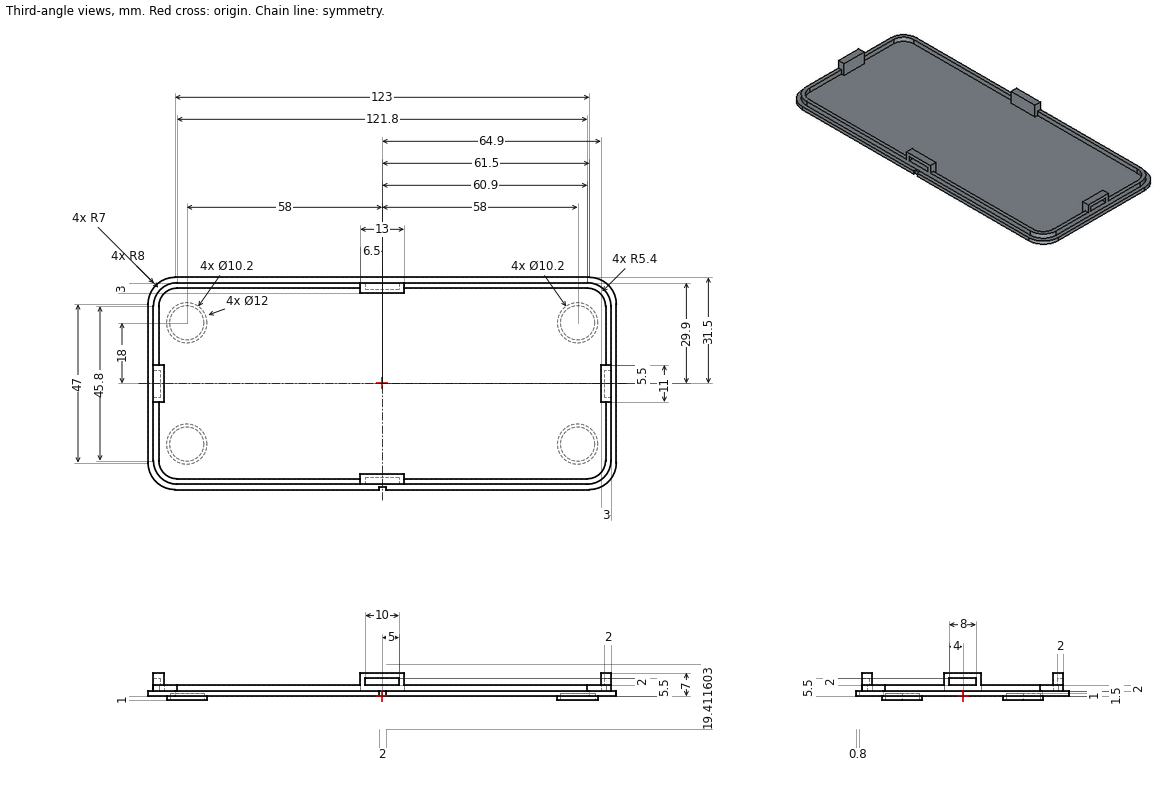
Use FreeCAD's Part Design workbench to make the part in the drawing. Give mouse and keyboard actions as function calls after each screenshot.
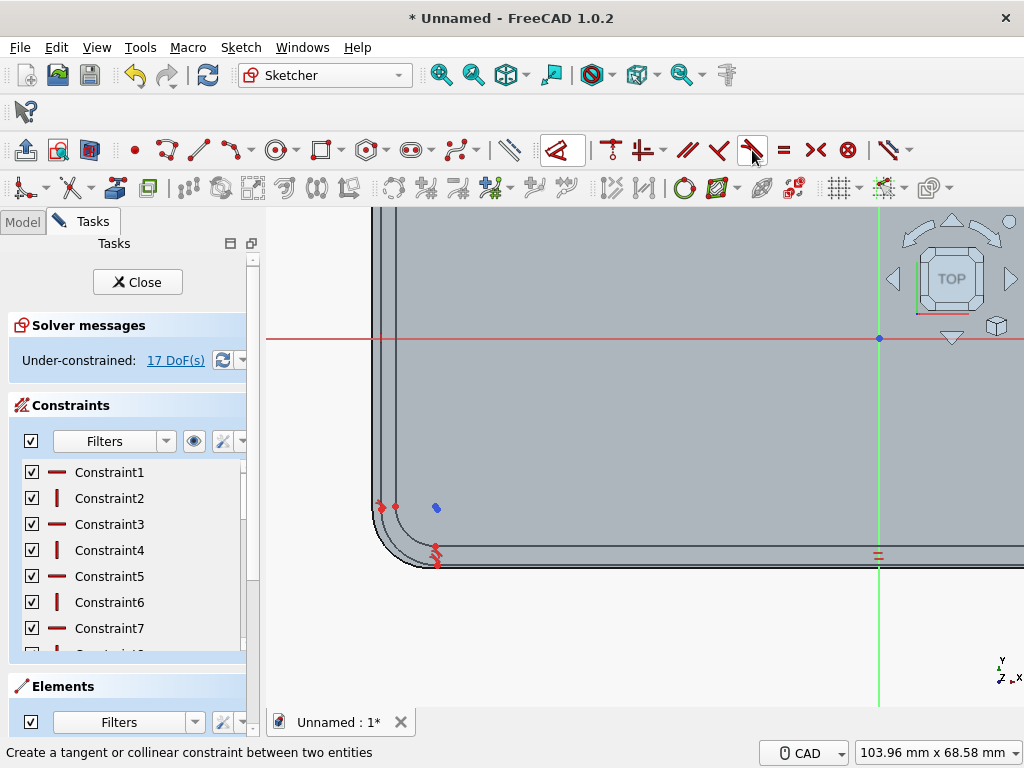
click(396, 406)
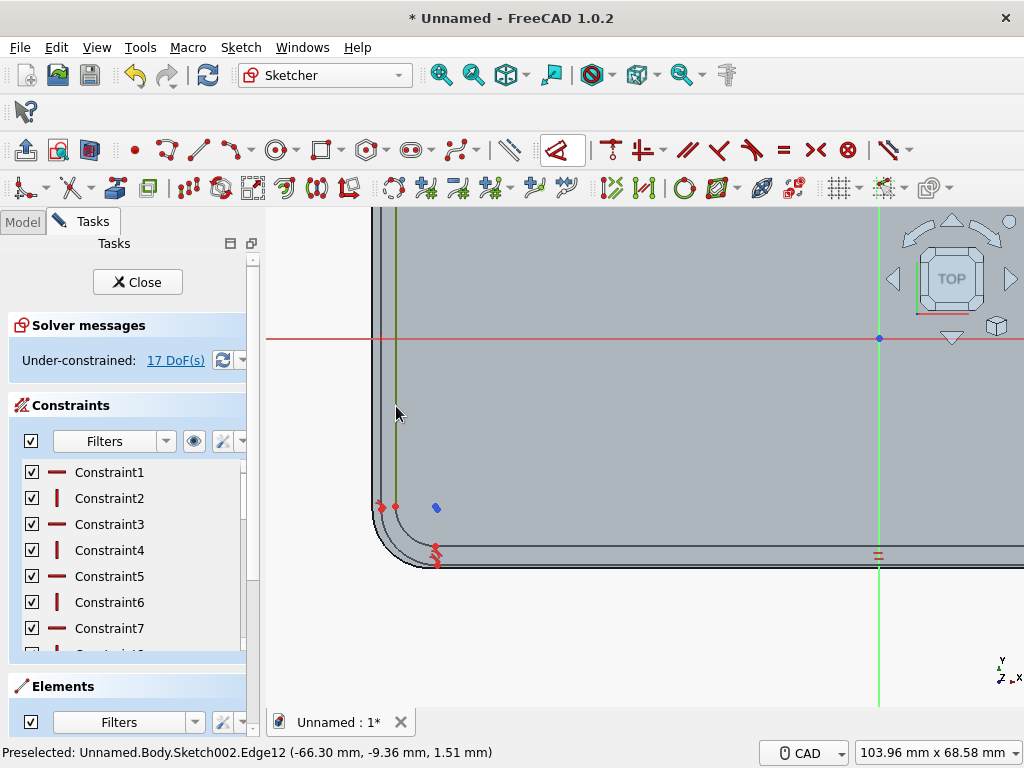
scroll(400, 526, down, 5)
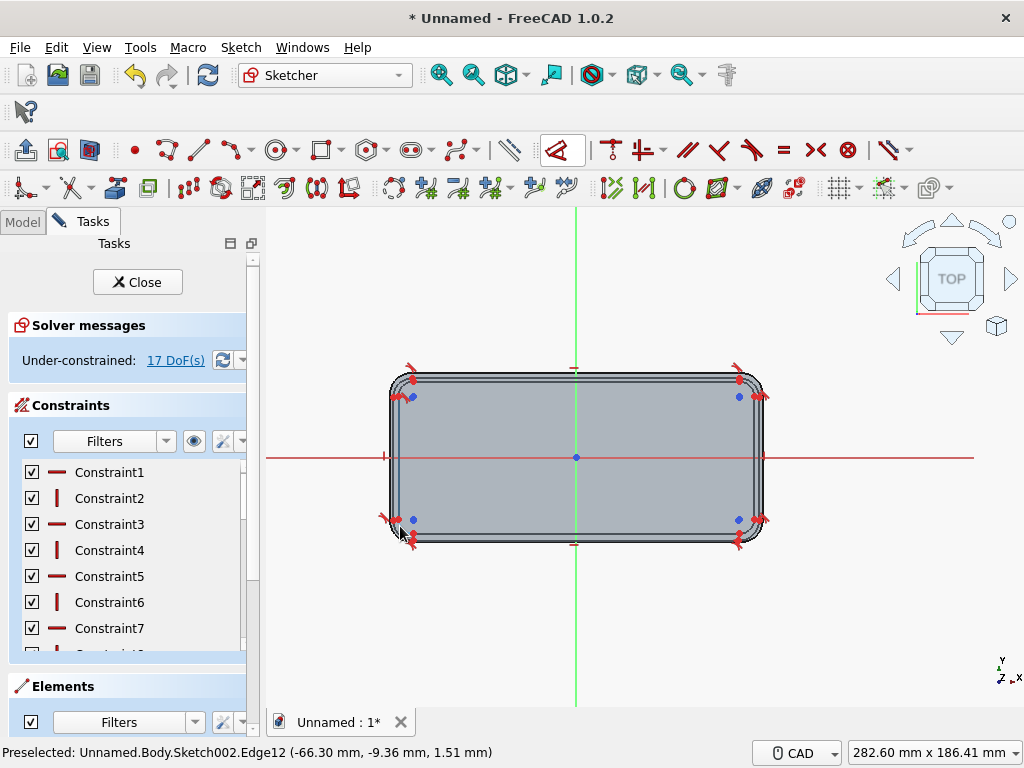
scroll(406, 383, up, 7)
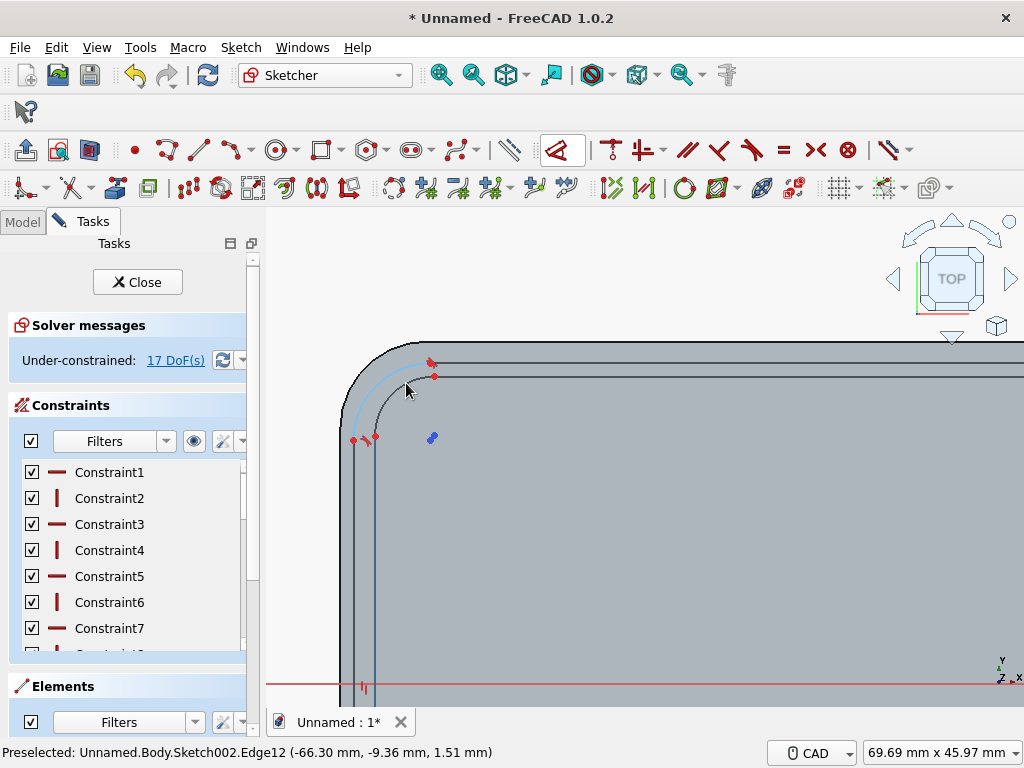
click(407, 383)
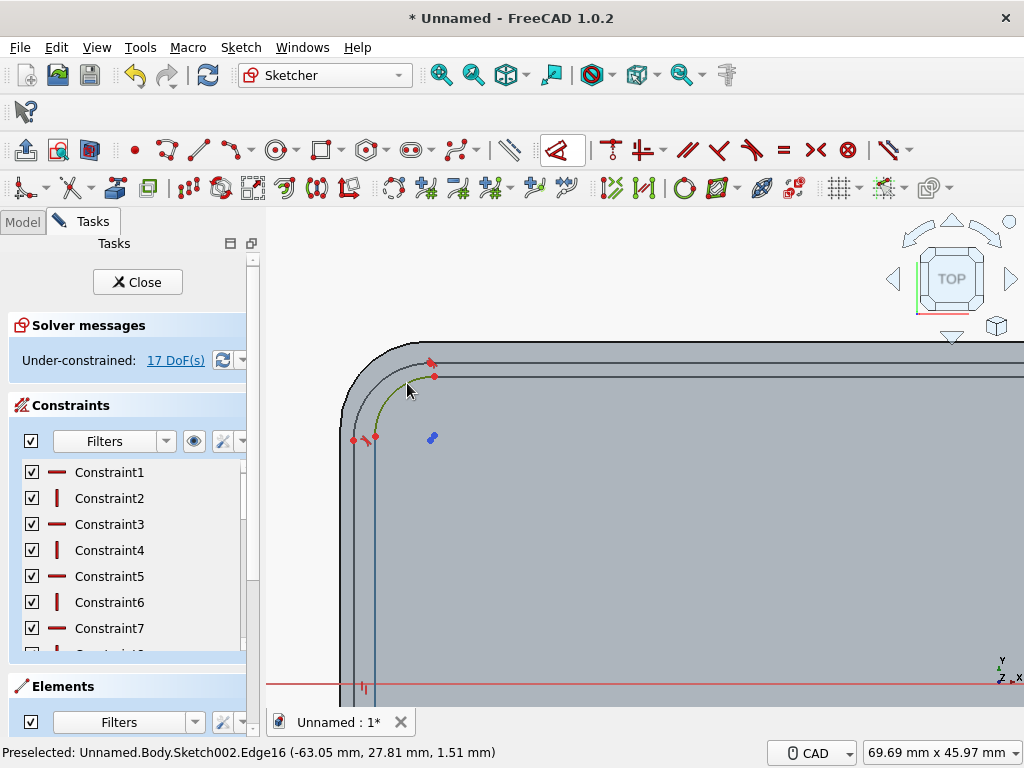
click(752, 150)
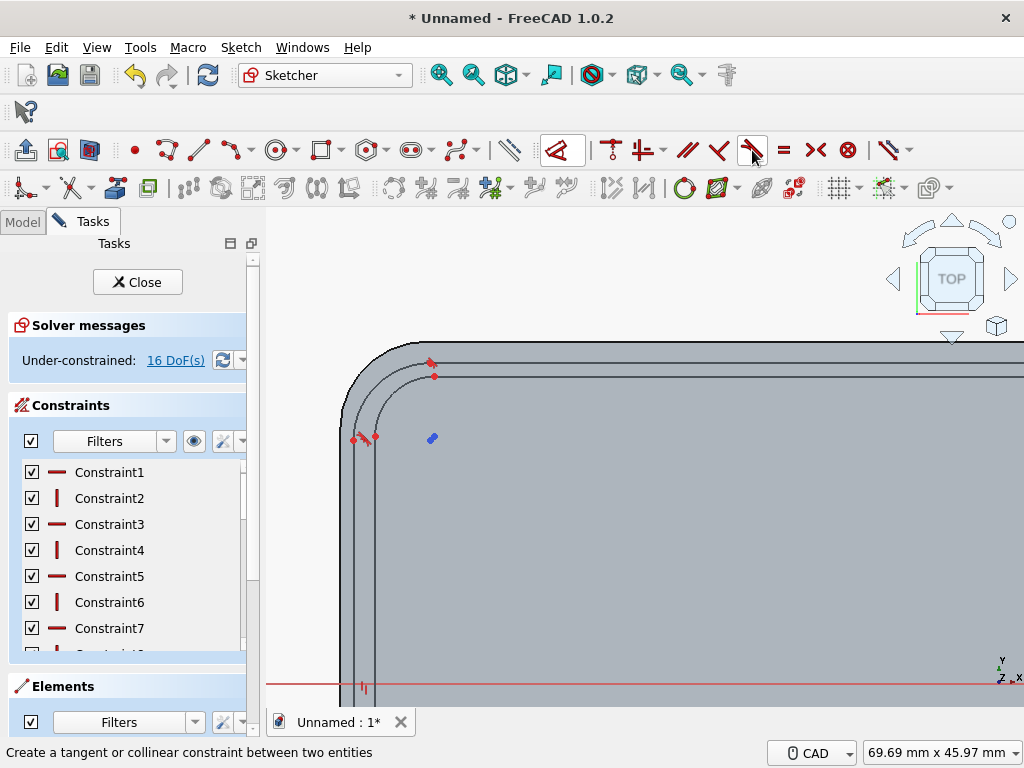
scroll(406, 383, down, 7)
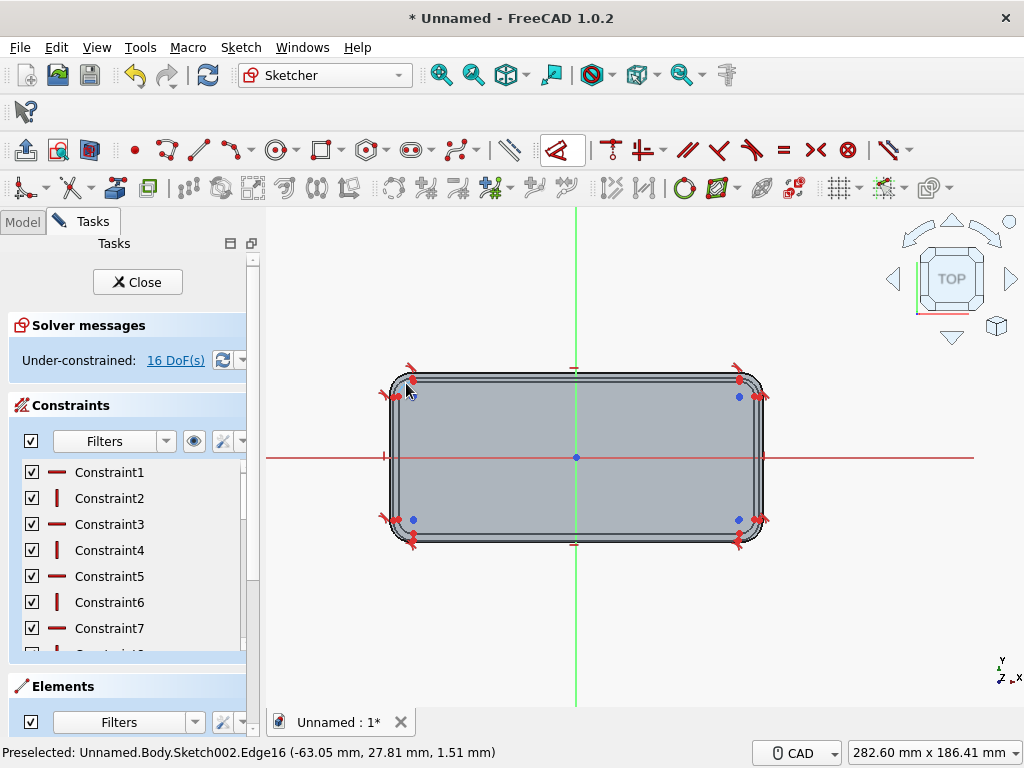
scroll(757, 389, up, 6)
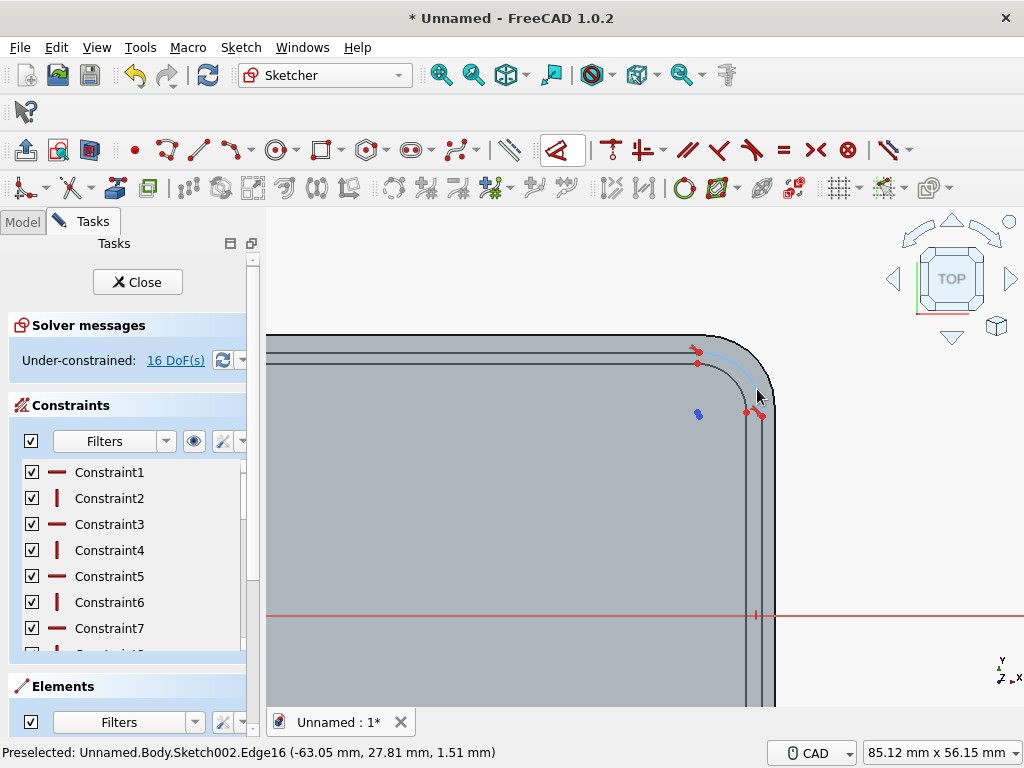
click(755, 387)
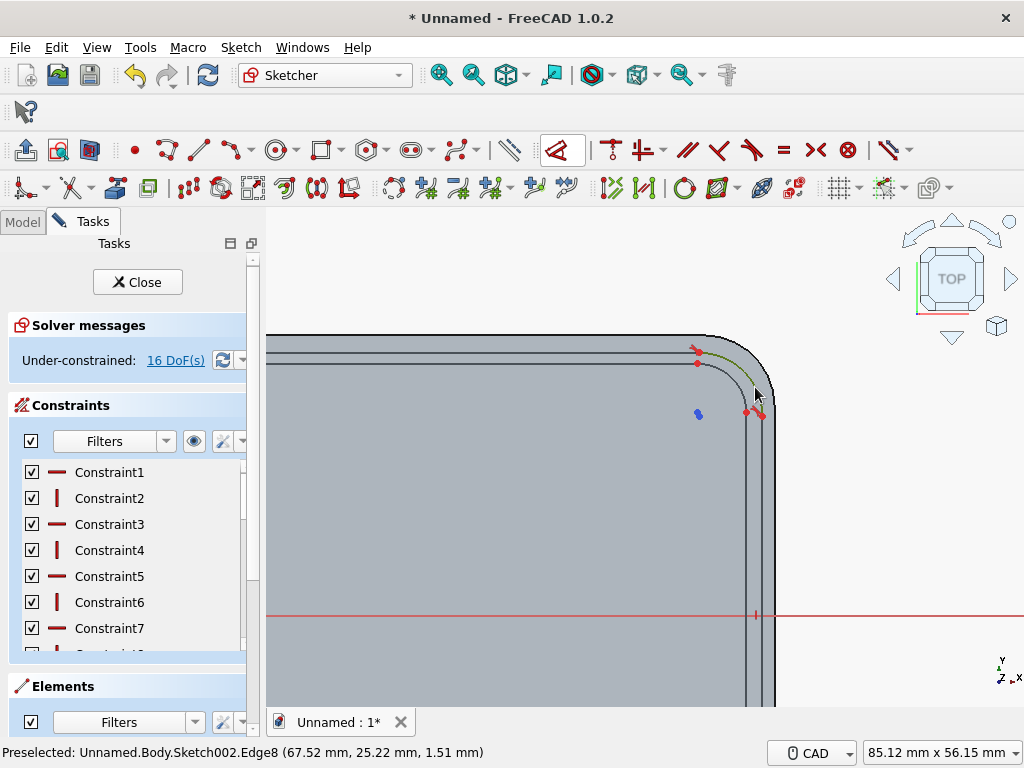
click(741, 390)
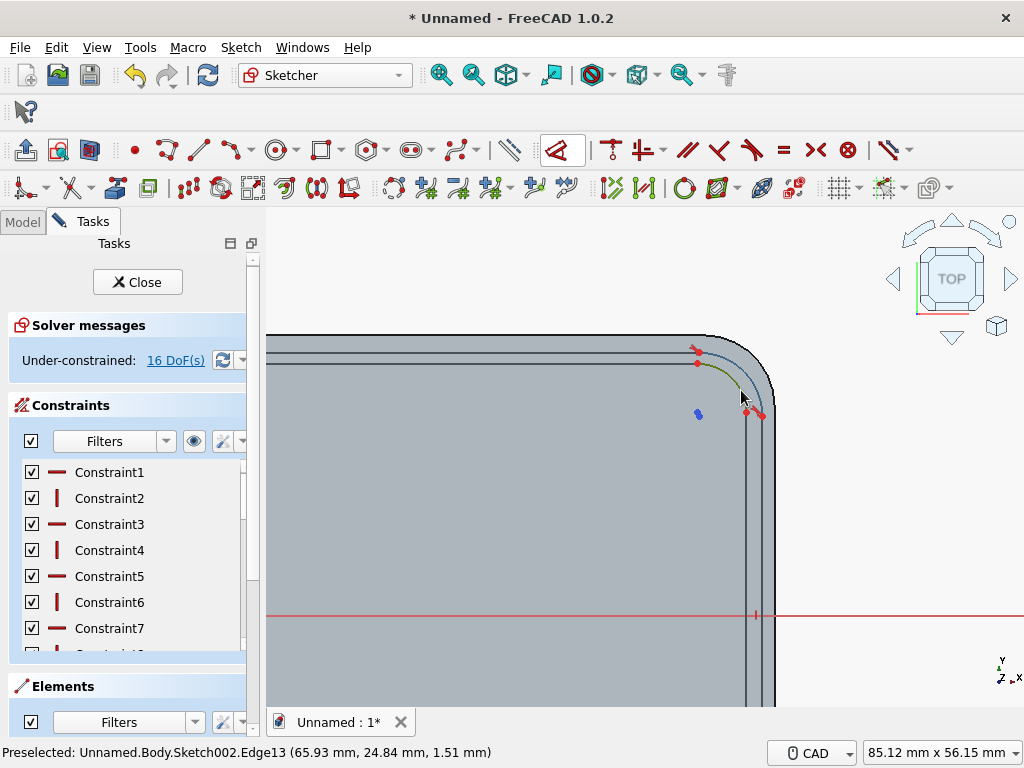
click(612, 150)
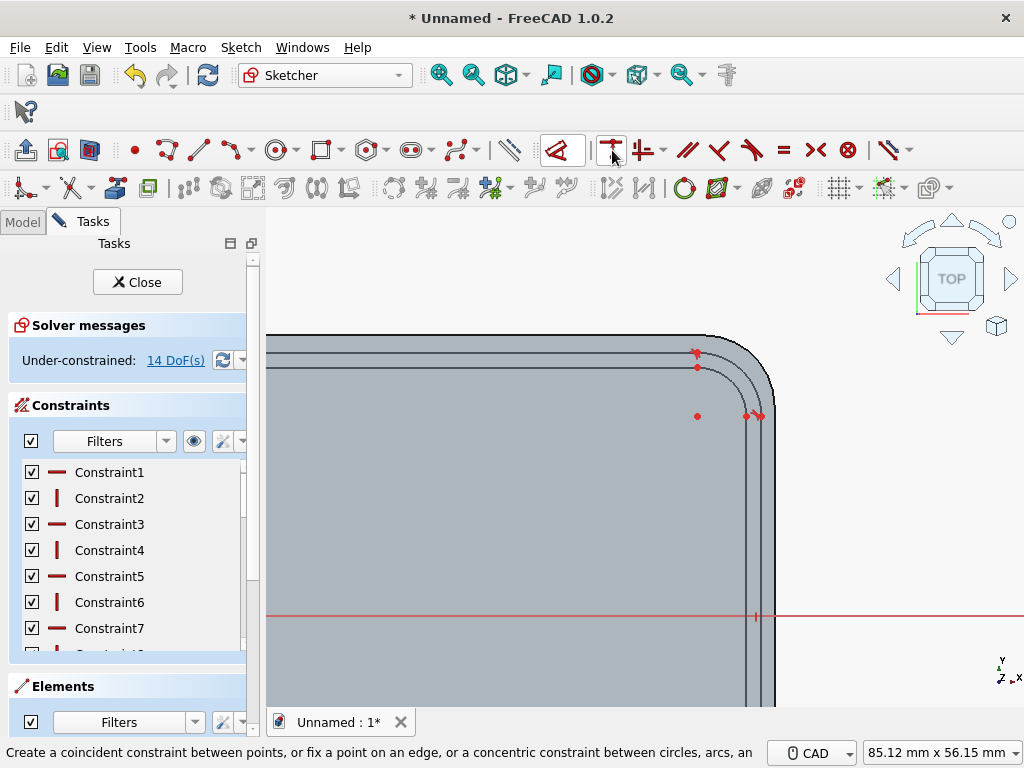
scroll(758, 389, down, 6)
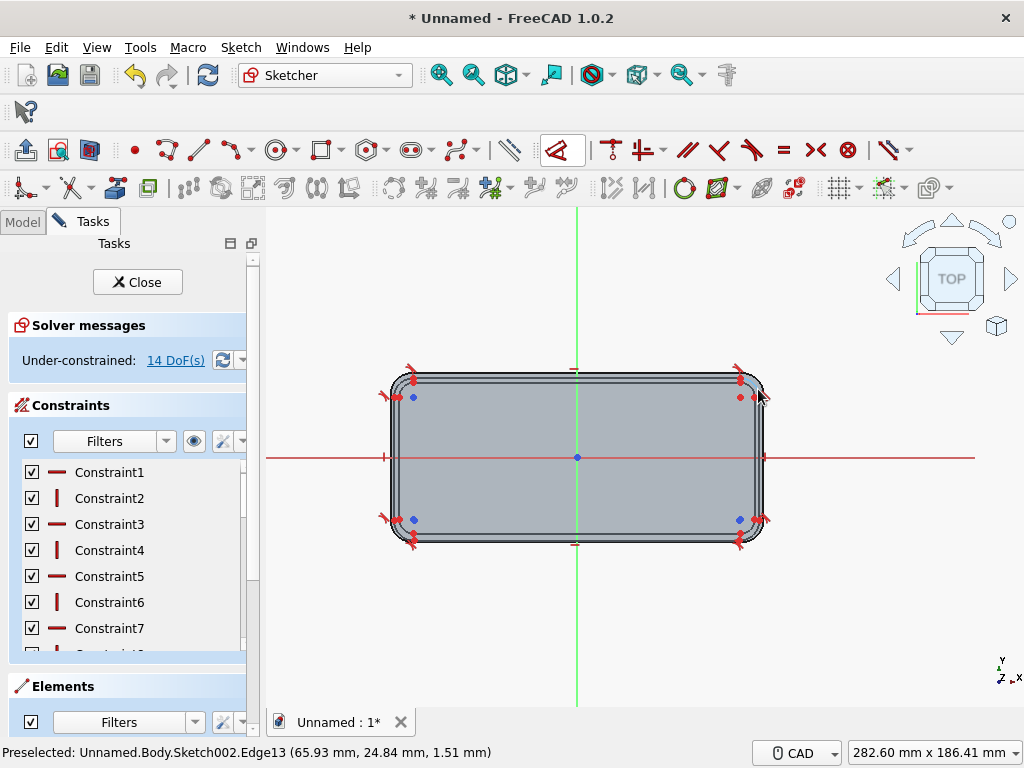
scroll(748, 539, up, 4)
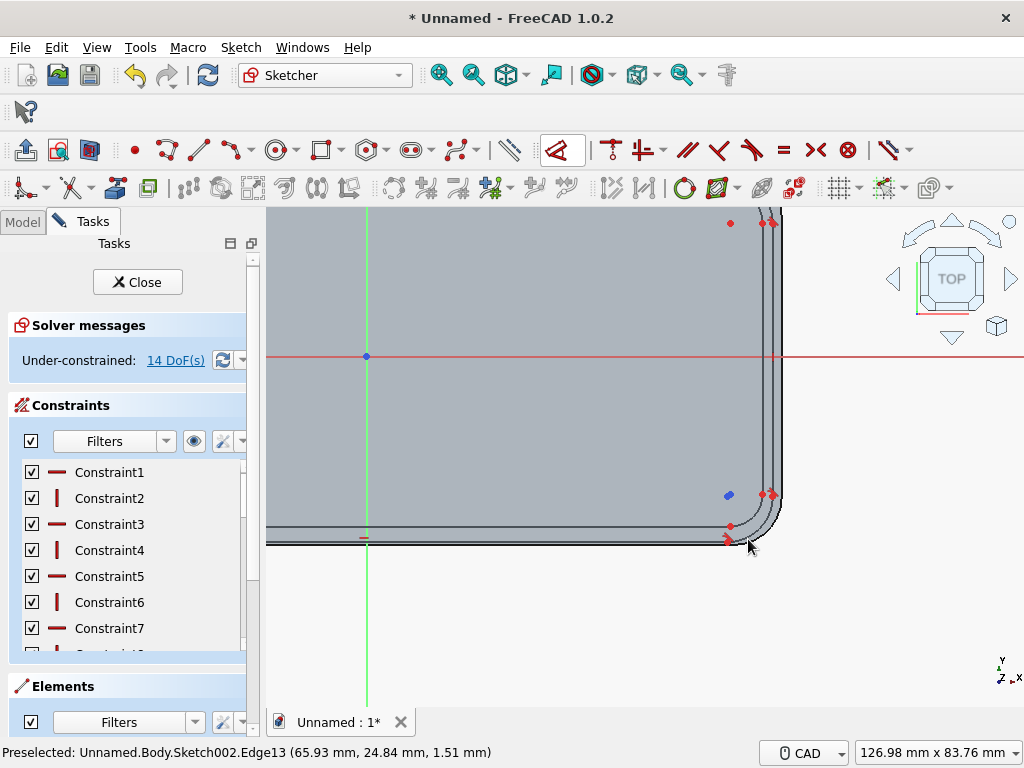
click(748, 537)